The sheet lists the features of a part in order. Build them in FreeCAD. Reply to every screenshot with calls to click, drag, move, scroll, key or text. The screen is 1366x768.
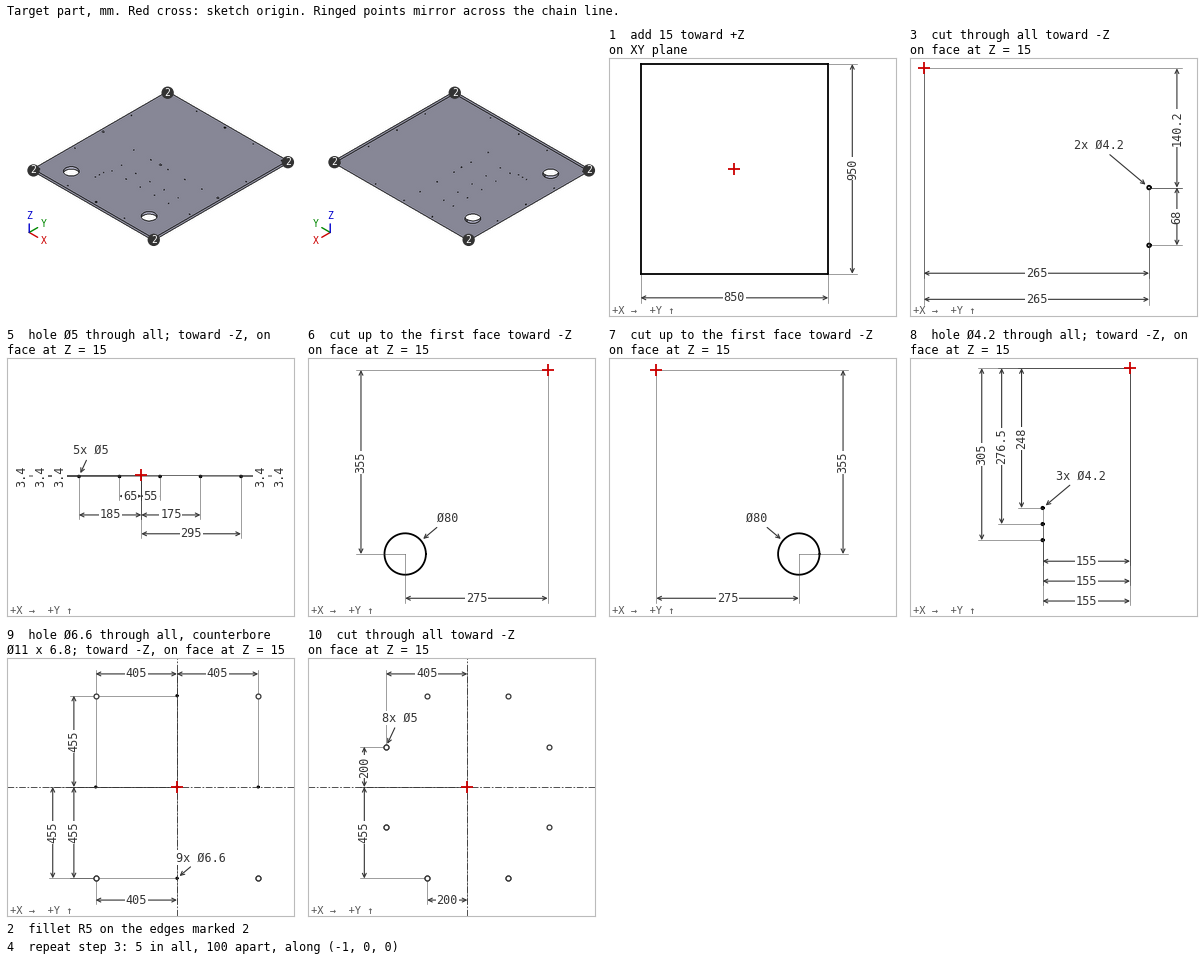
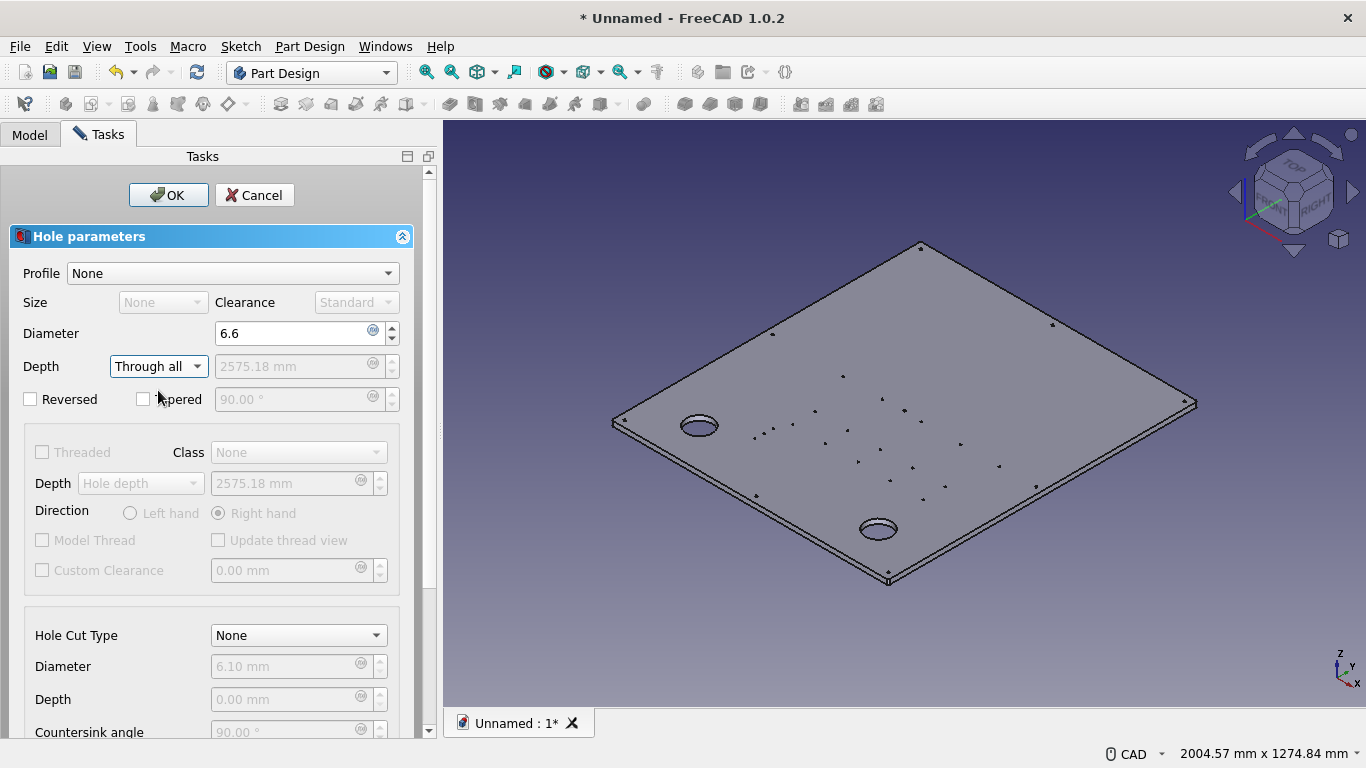
click(300, 636)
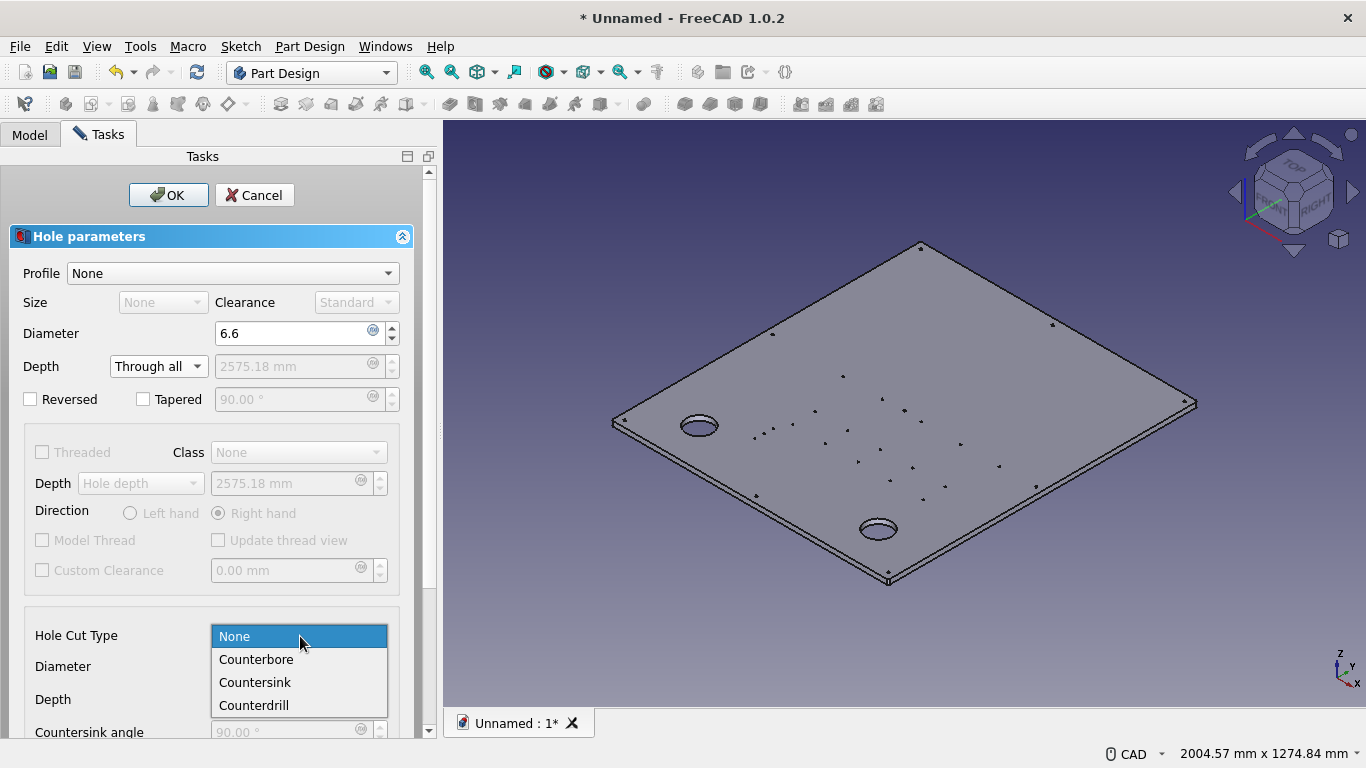
click(298, 660)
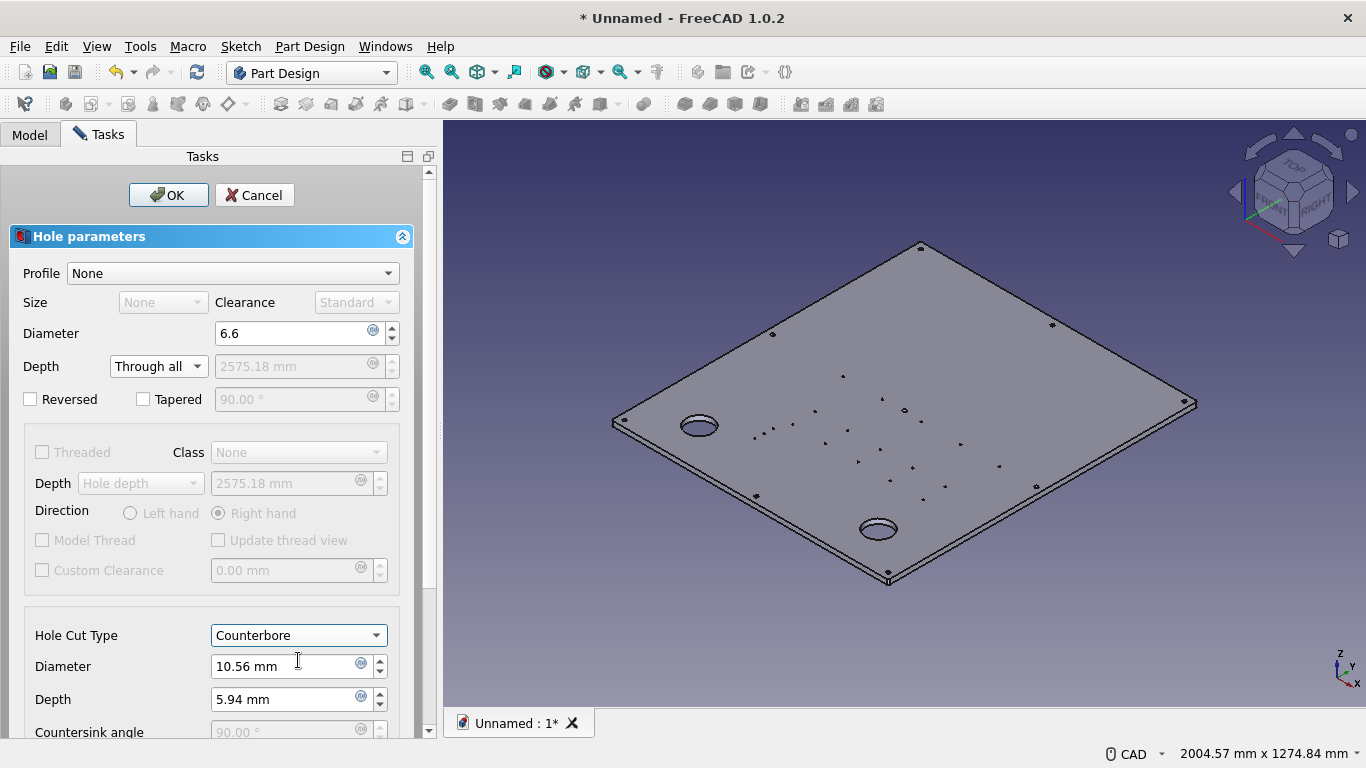
triple_click(292, 666)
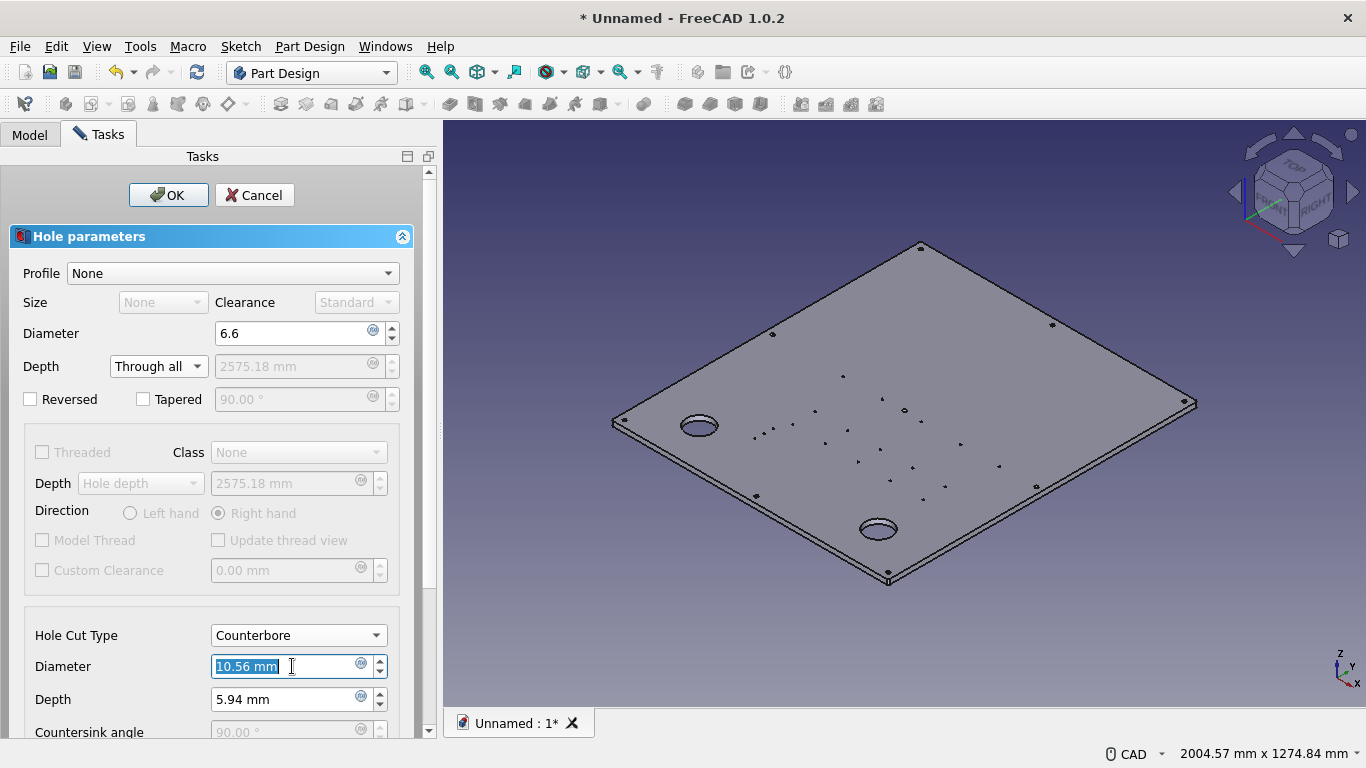
text(11)
key(Tab)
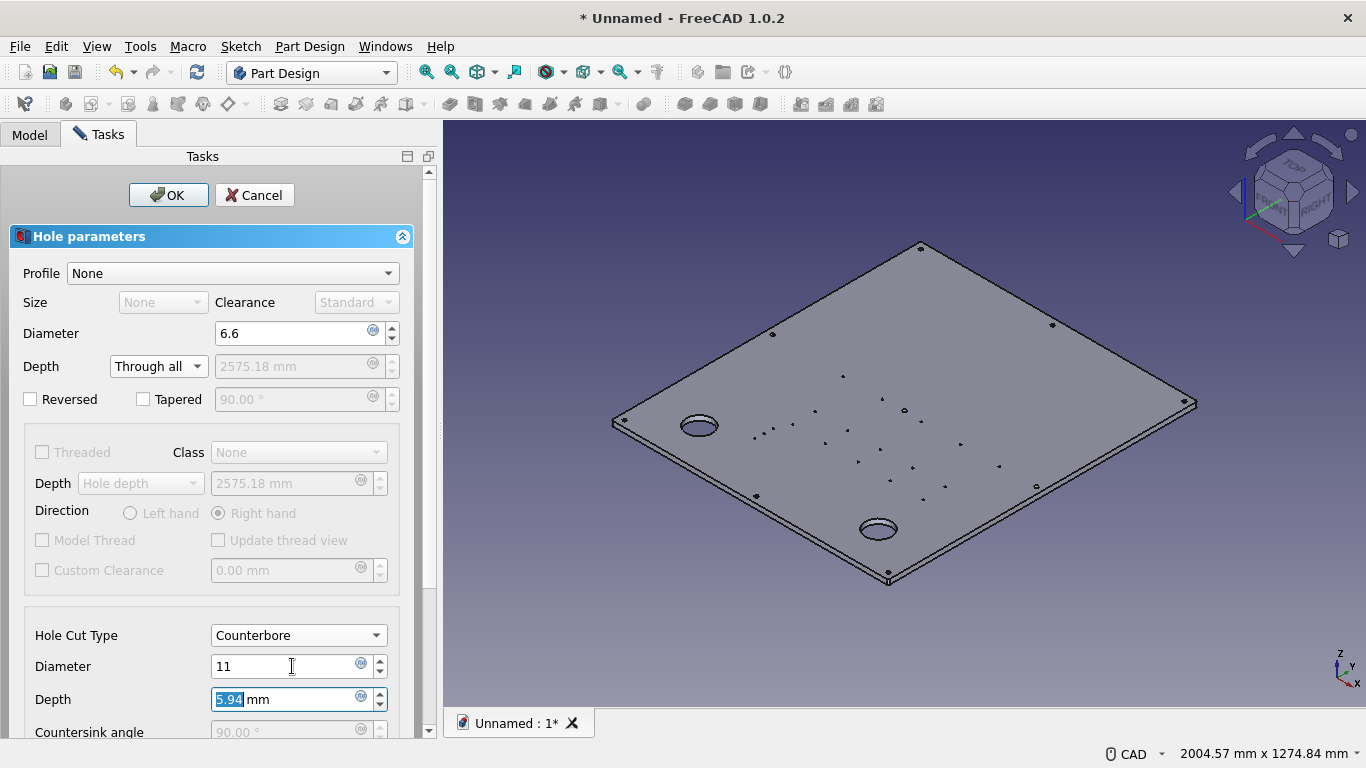
text(6.8)
key(Tab)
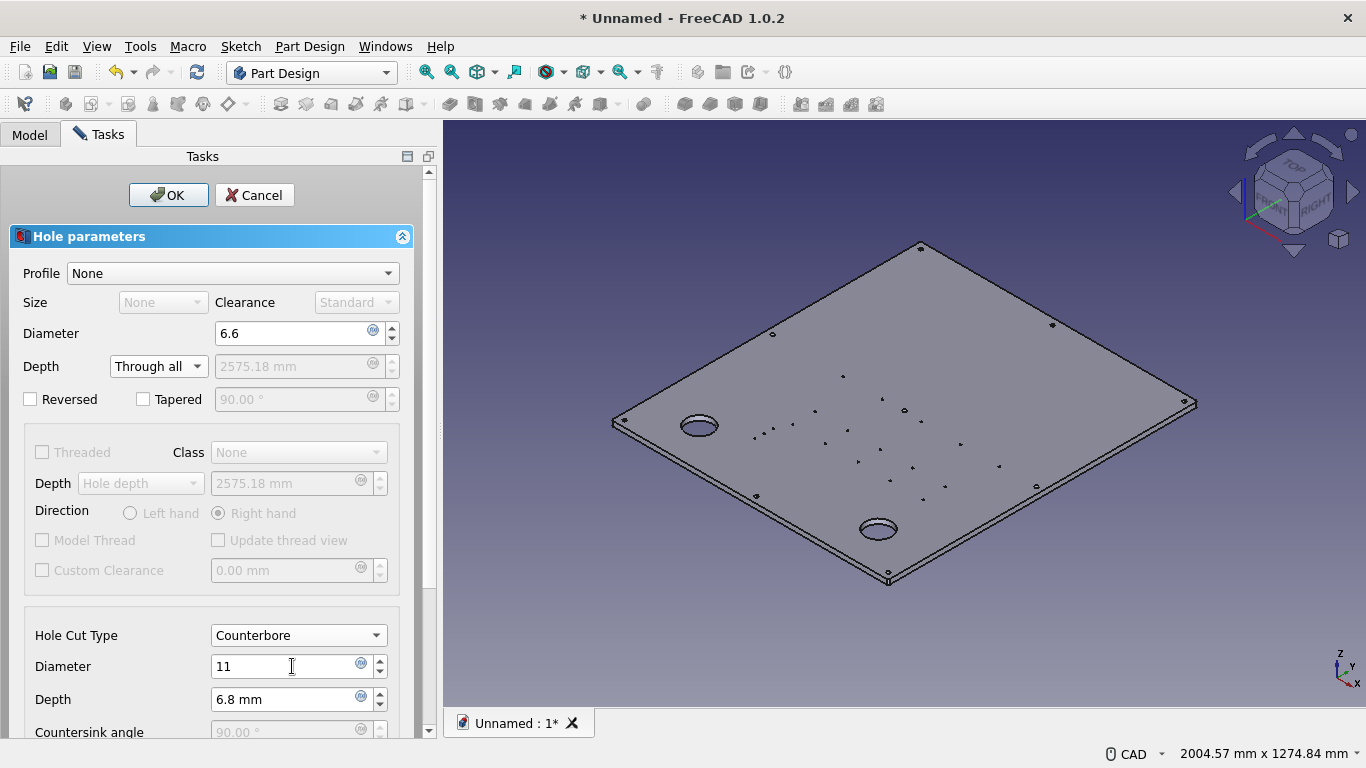
click(169, 195)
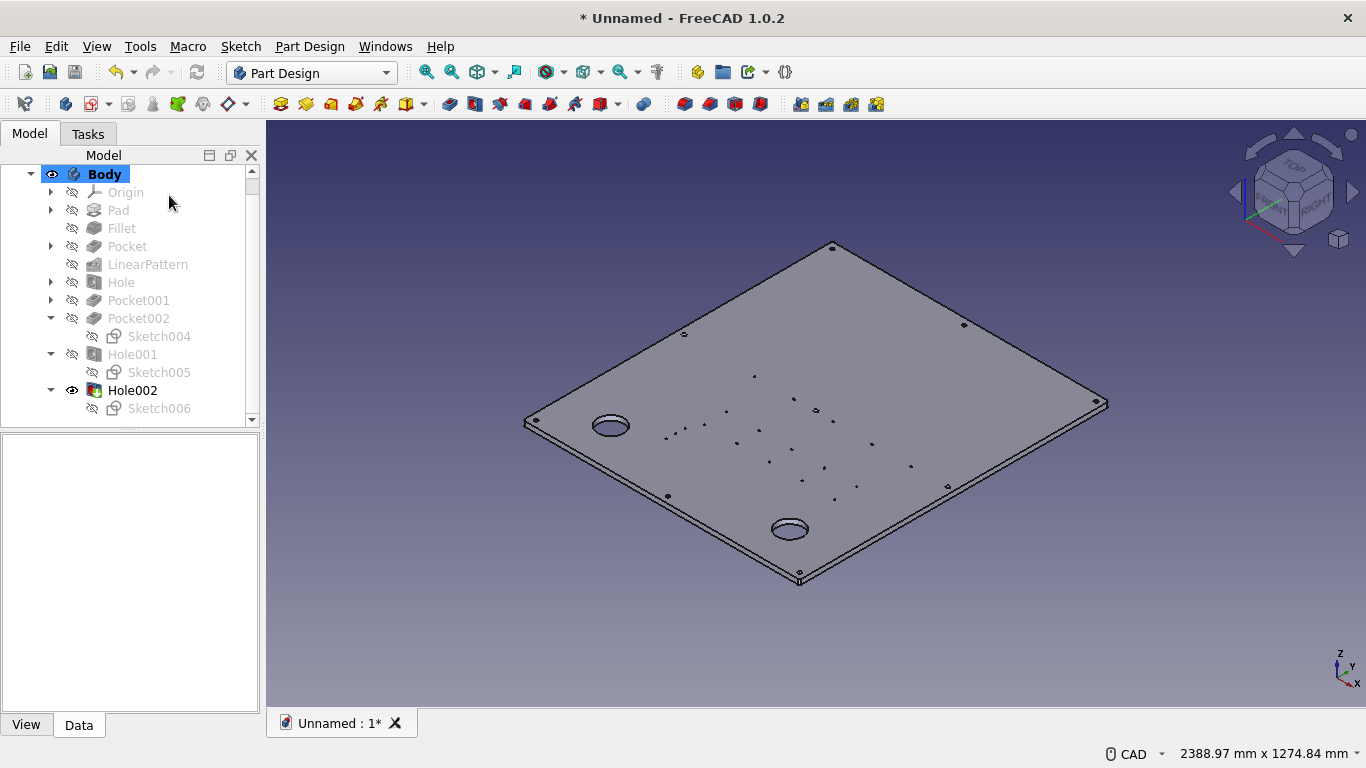
click(944, 381)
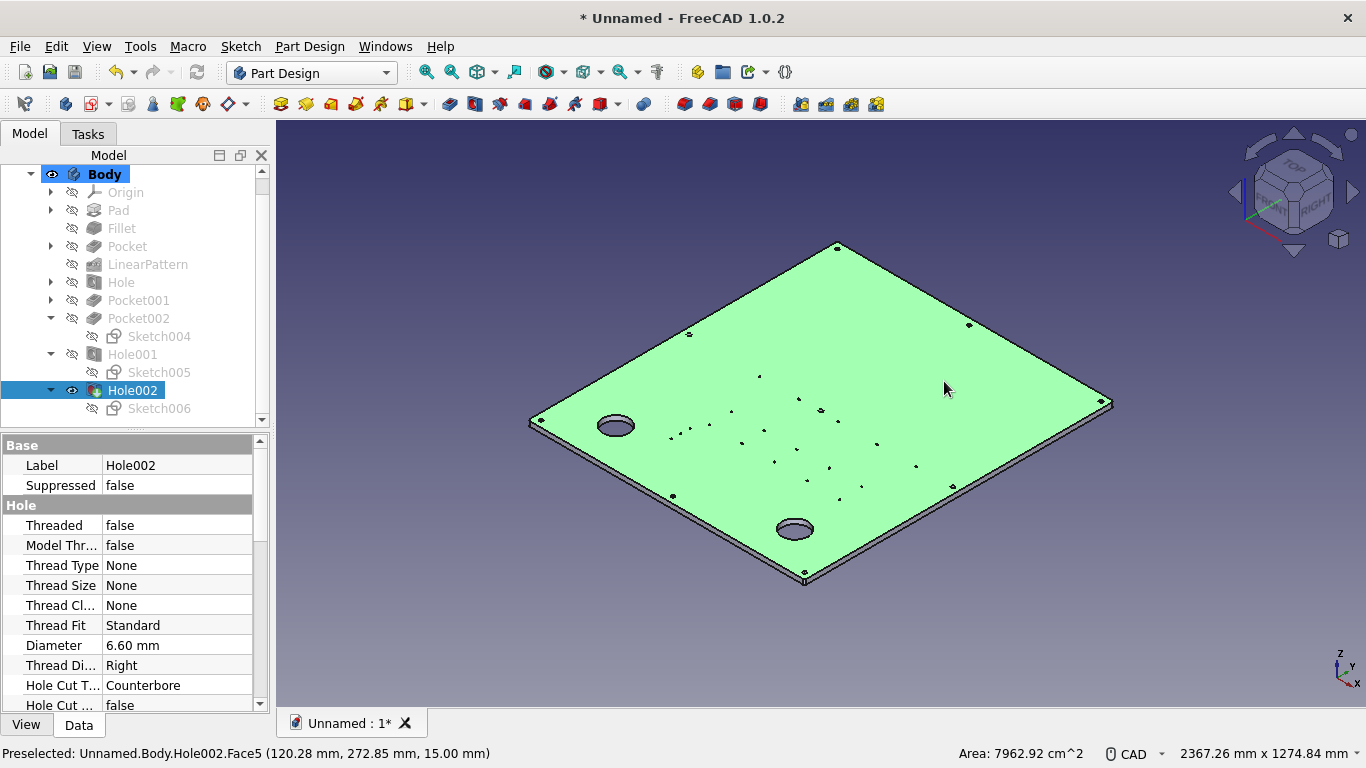
click(90, 104)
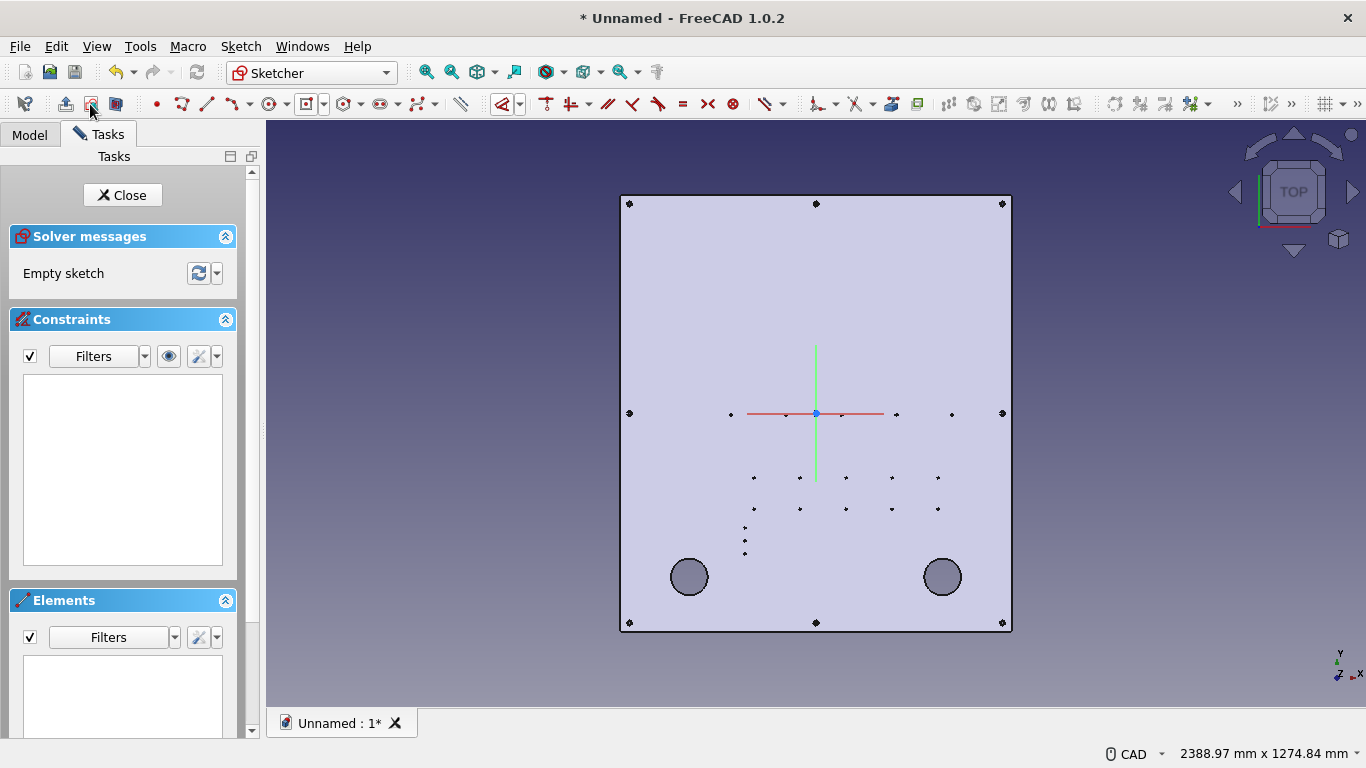
click(268, 104)